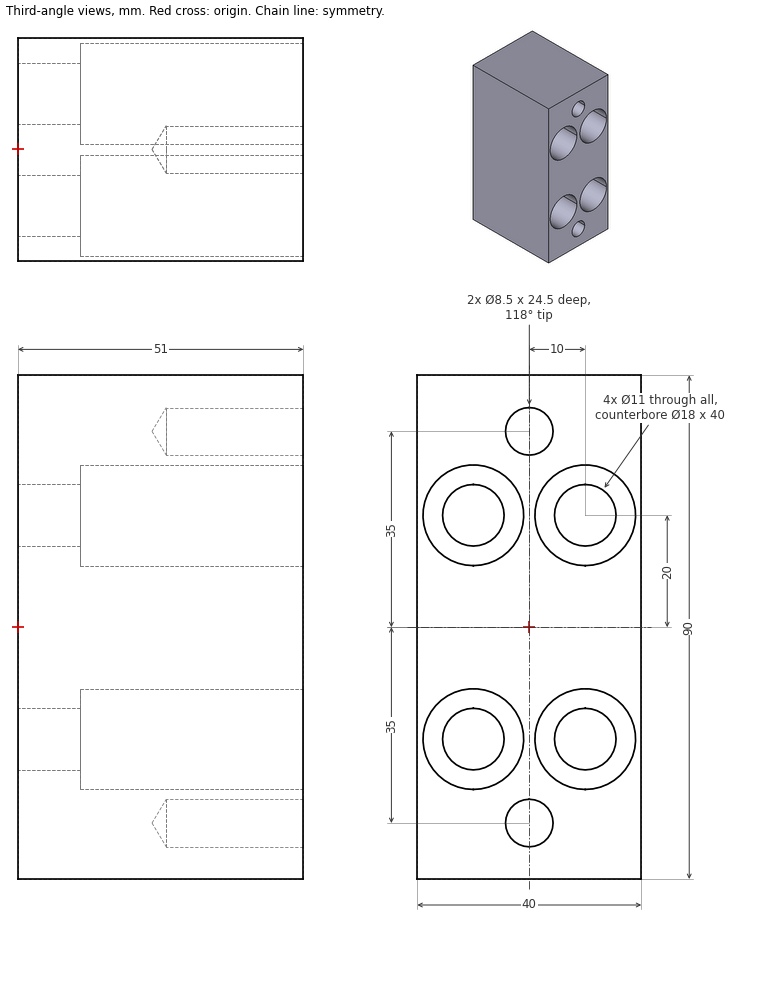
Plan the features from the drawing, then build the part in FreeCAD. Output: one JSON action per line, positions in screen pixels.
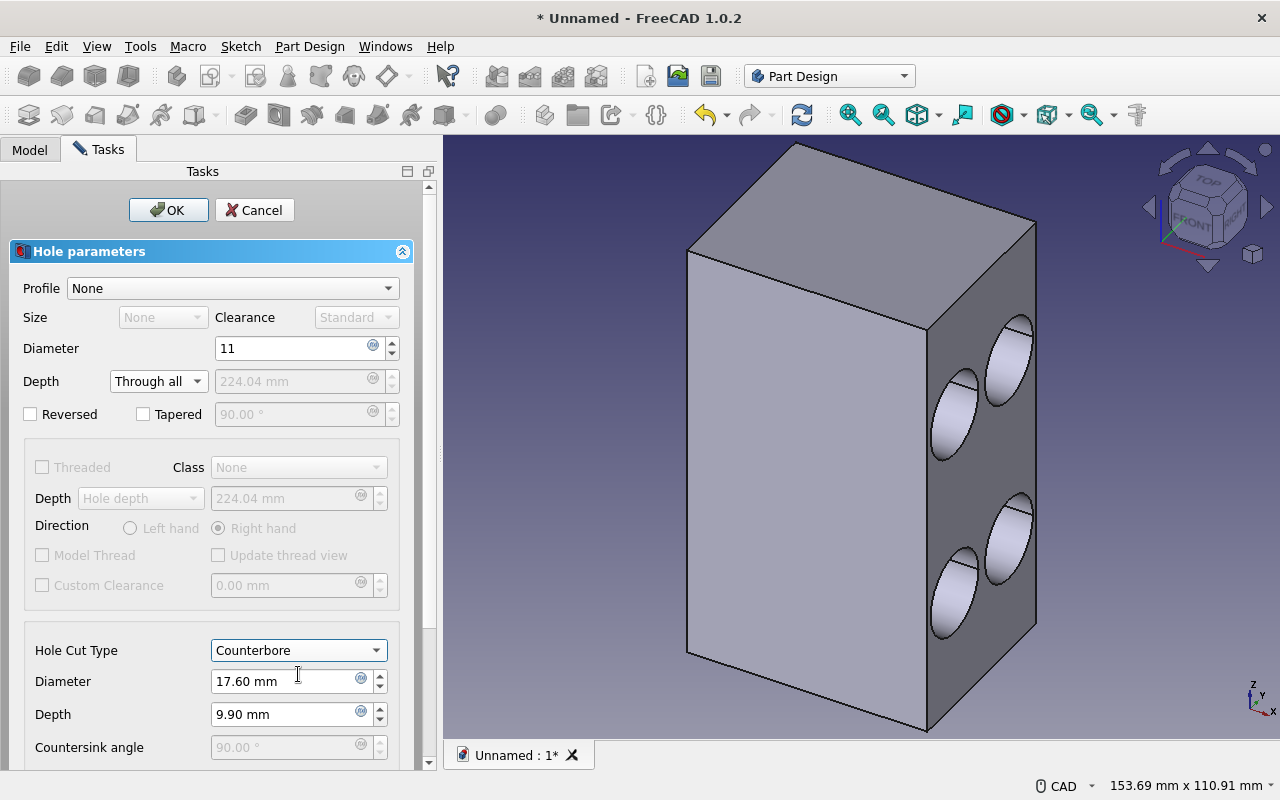
{"action": "triple_click", "coordinate": [292, 682]}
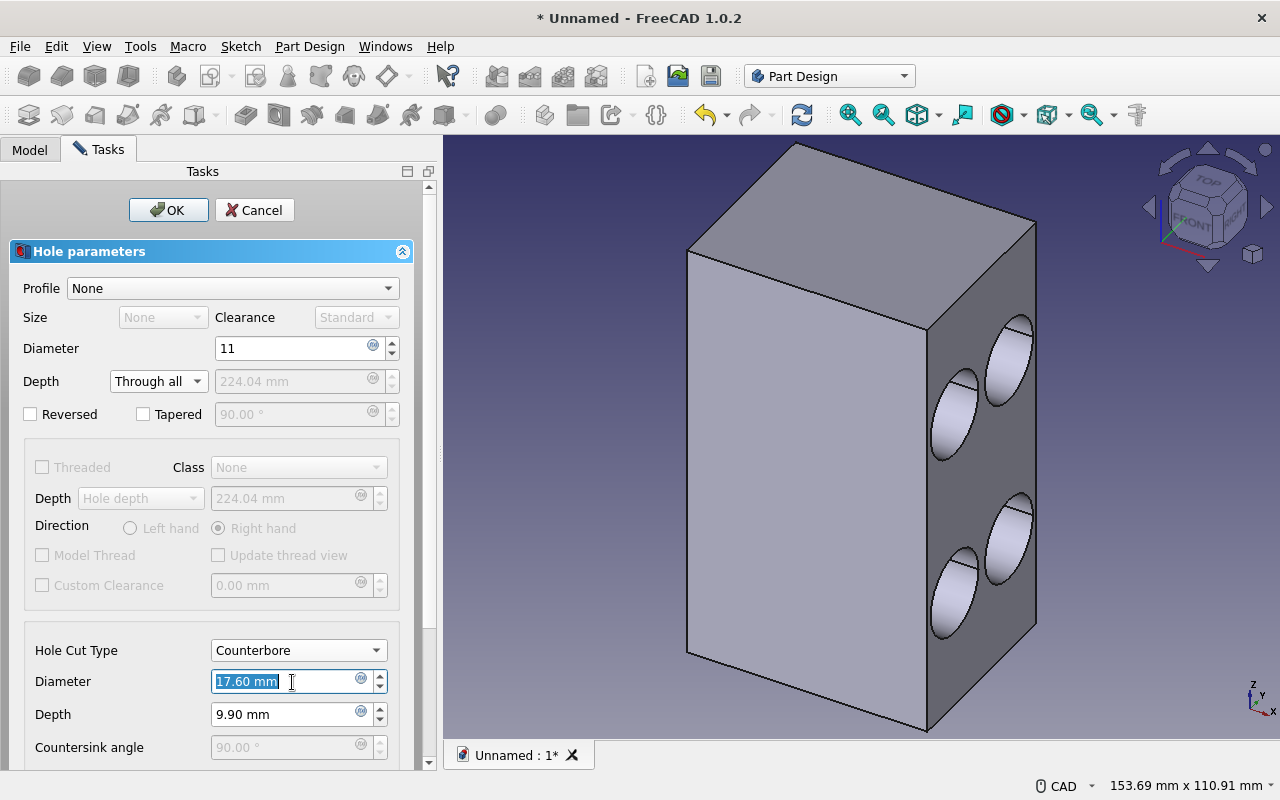
{"action": "type", "text": "18"}
{"action": "key", "text": "Tab"}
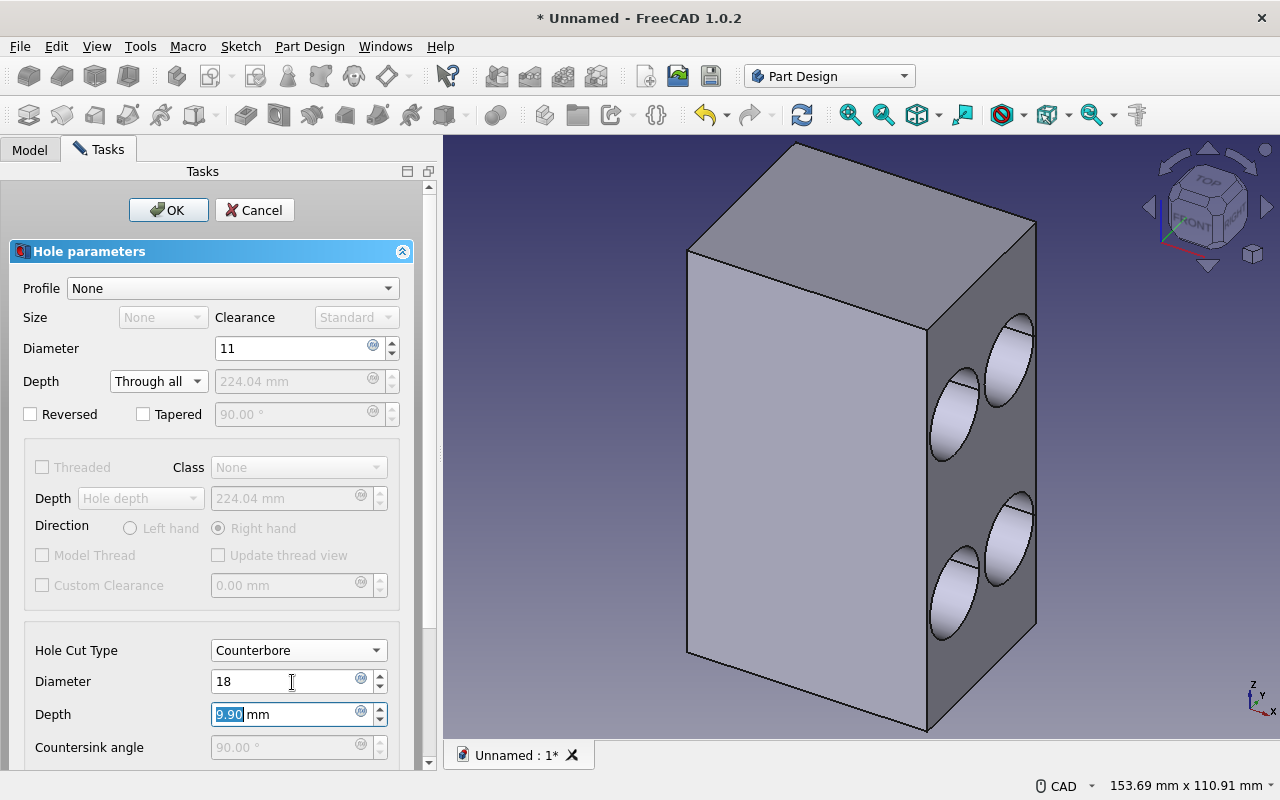
{"action": "type", "text": "40"}
{"action": "key", "text": "Tab"}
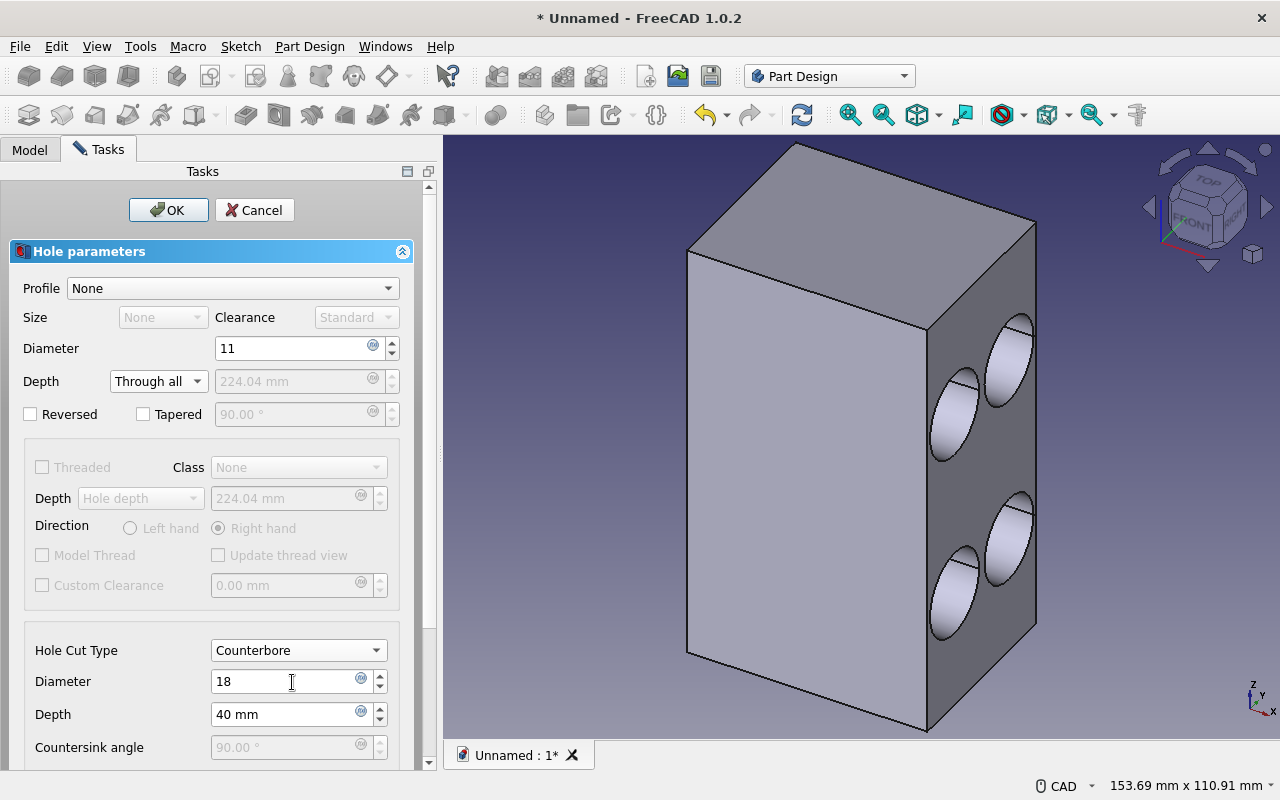
{"action": "left_click", "coordinate": [169, 210]}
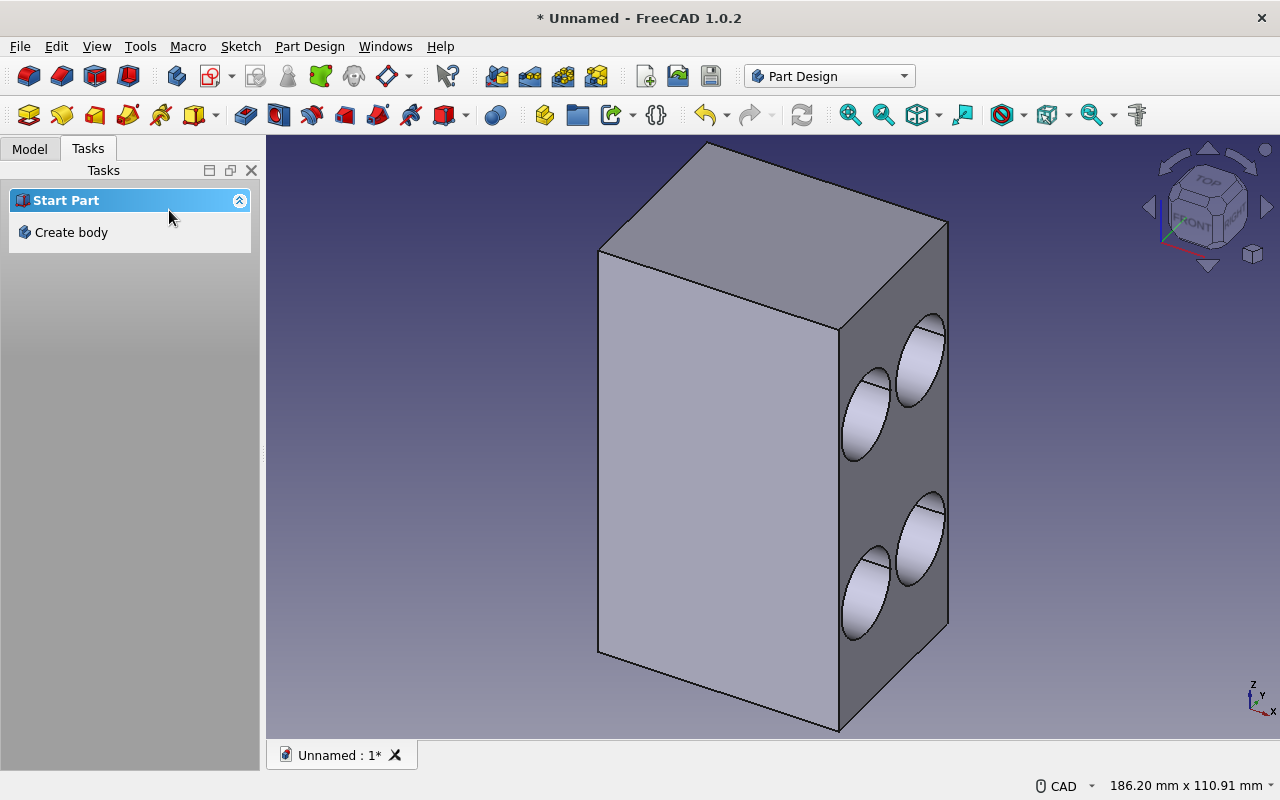
{"action": "left_click", "coordinate": [893, 476]}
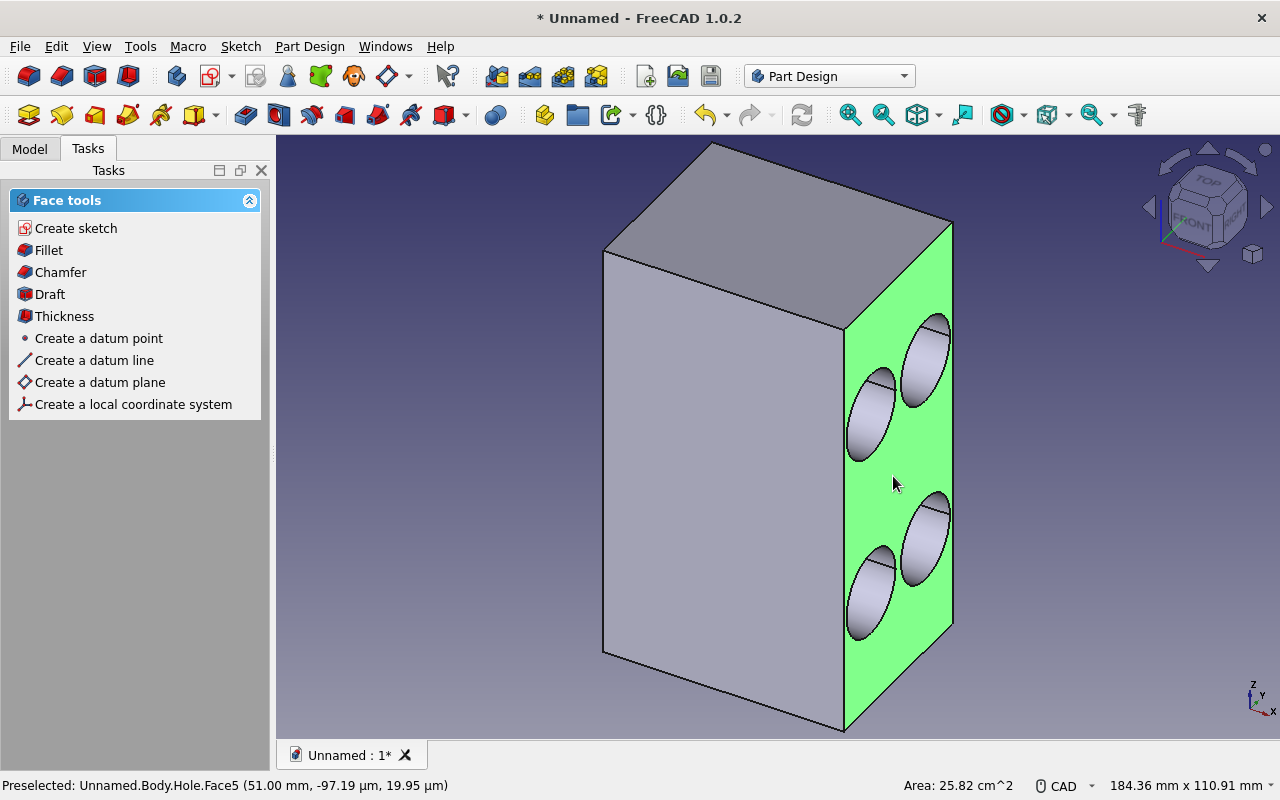
{"action": "left_click", "coordinate": [210, 76]}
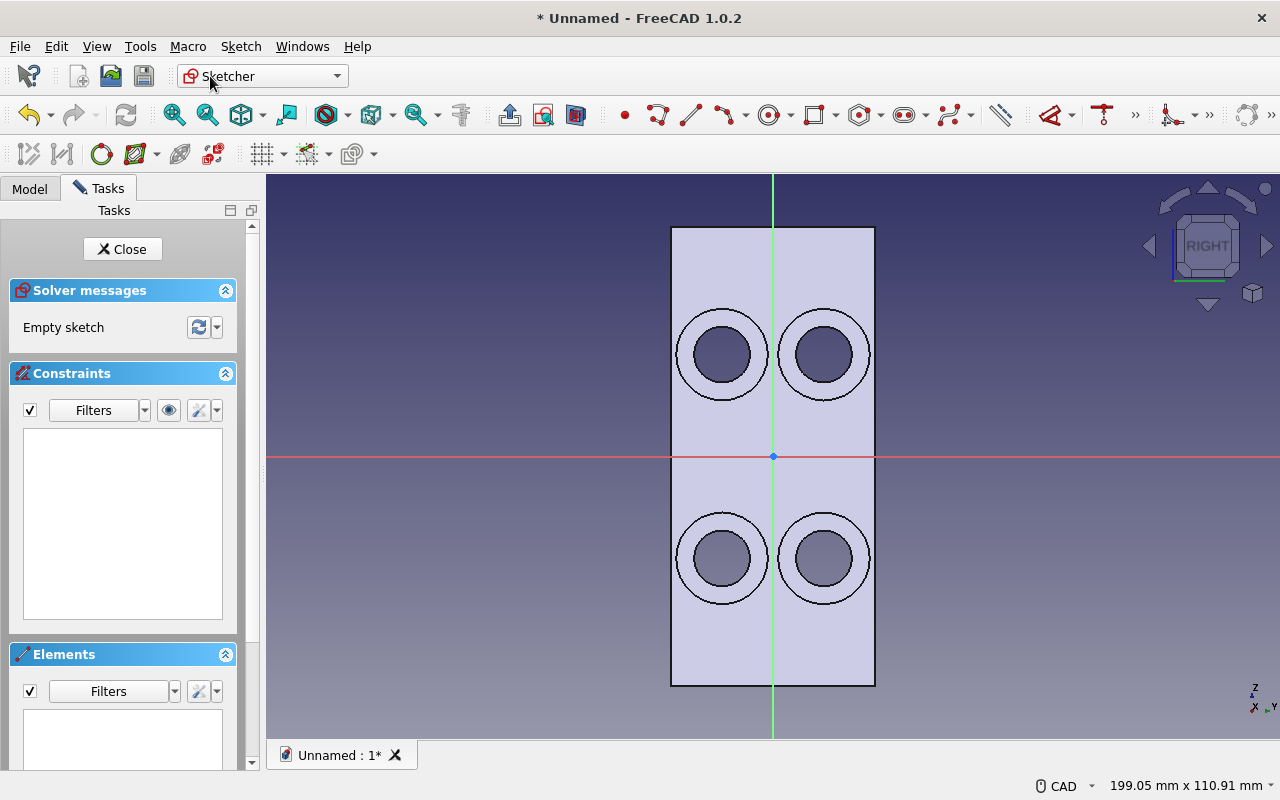
{"action": "left_click", "coordinate": [768, 116]}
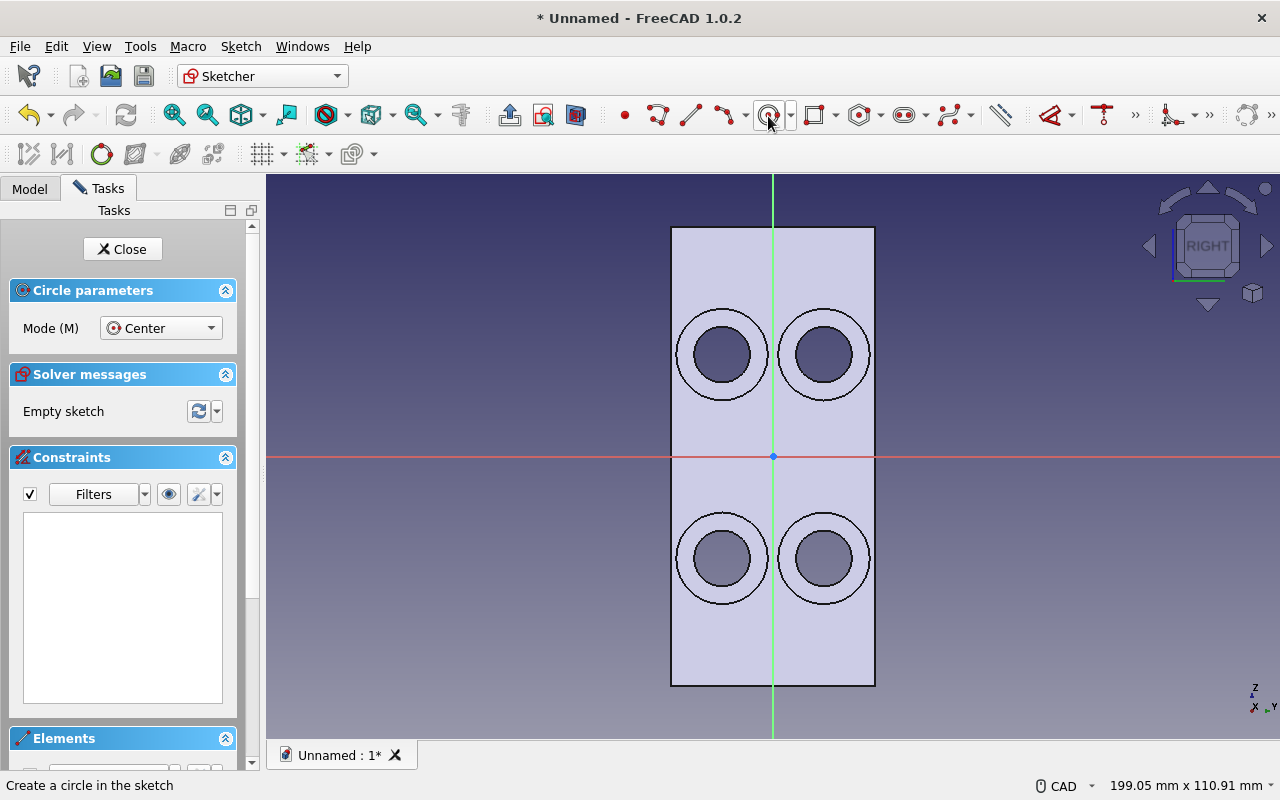
{"action": "left_click", "coordinate": [773, 278]}
{"action": "mouse_move", "coordinate": [788, 263]}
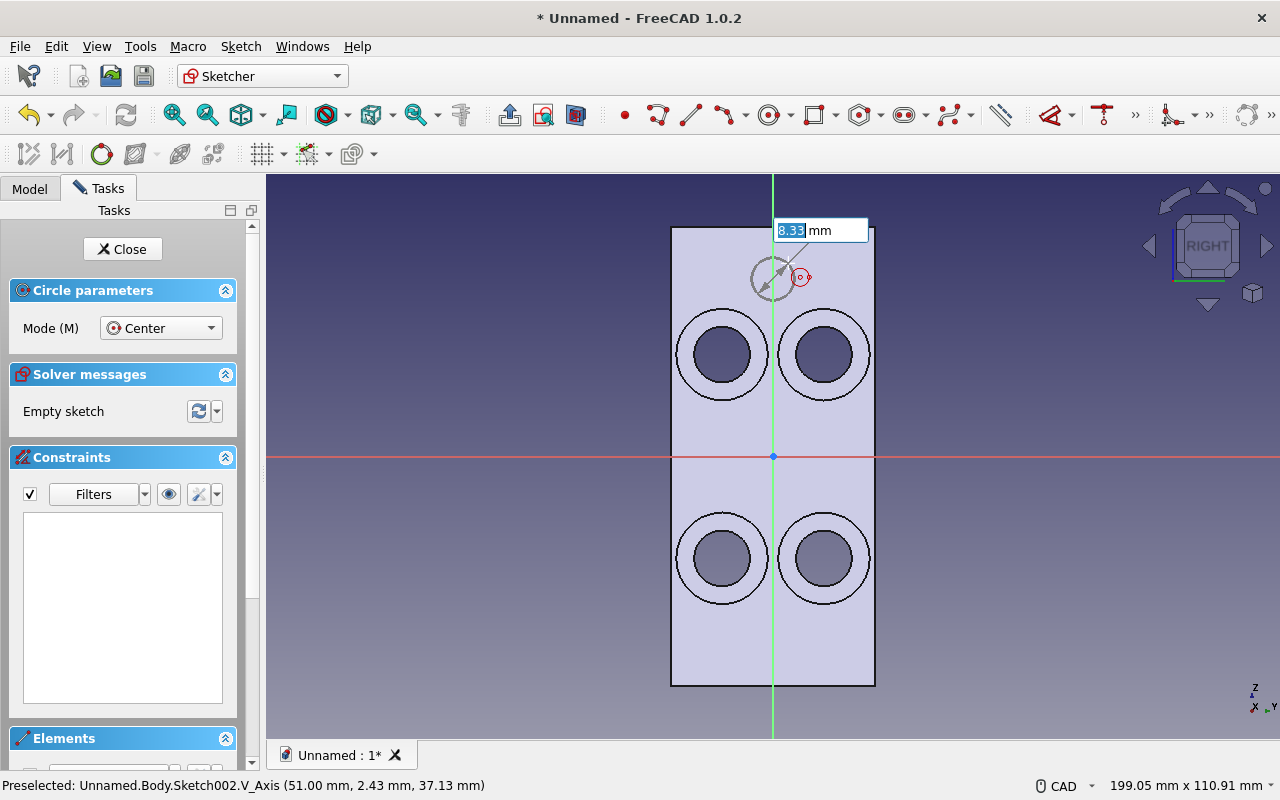
{"action": "type", "text": "8.5"}
{"action": "key", "text": "Return"}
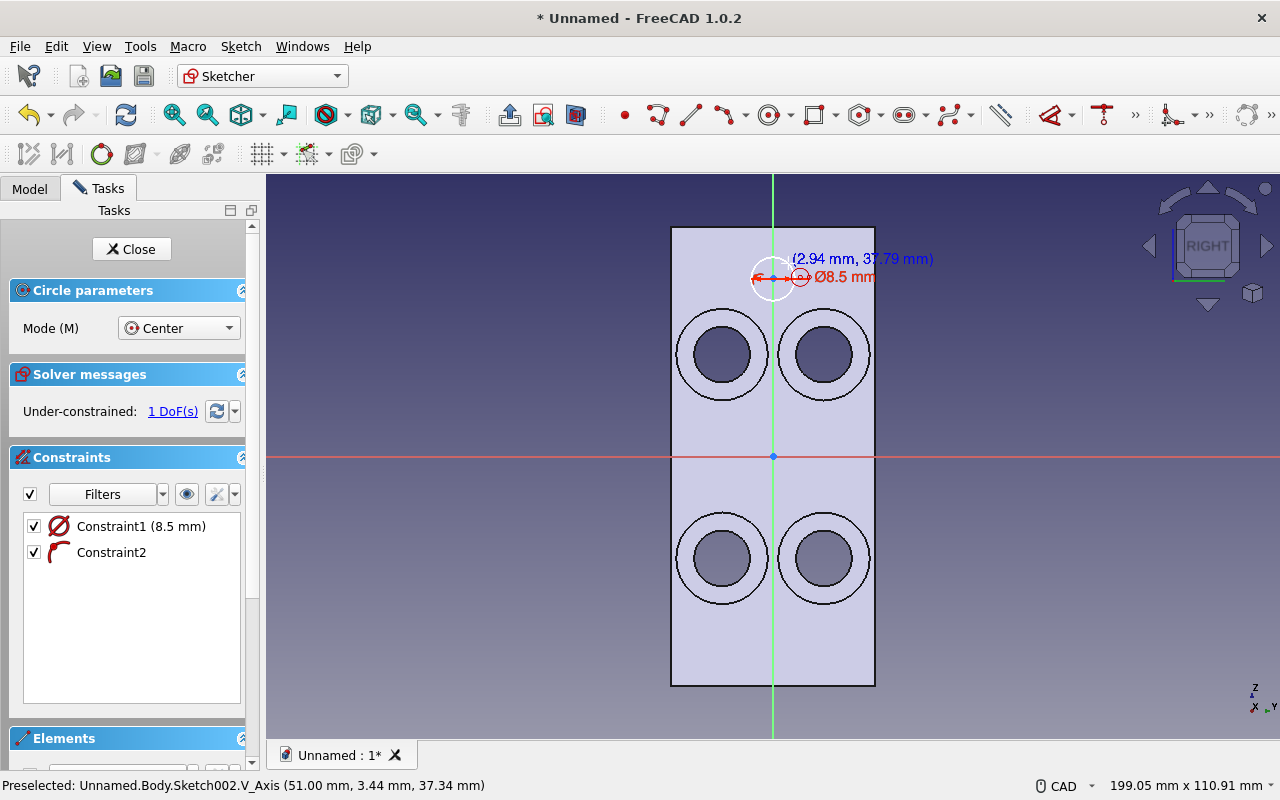
{"action": "left_click", "coordinate": [773, 635]}
{"action": "mouse_move", "coordinate": [788, 619]}